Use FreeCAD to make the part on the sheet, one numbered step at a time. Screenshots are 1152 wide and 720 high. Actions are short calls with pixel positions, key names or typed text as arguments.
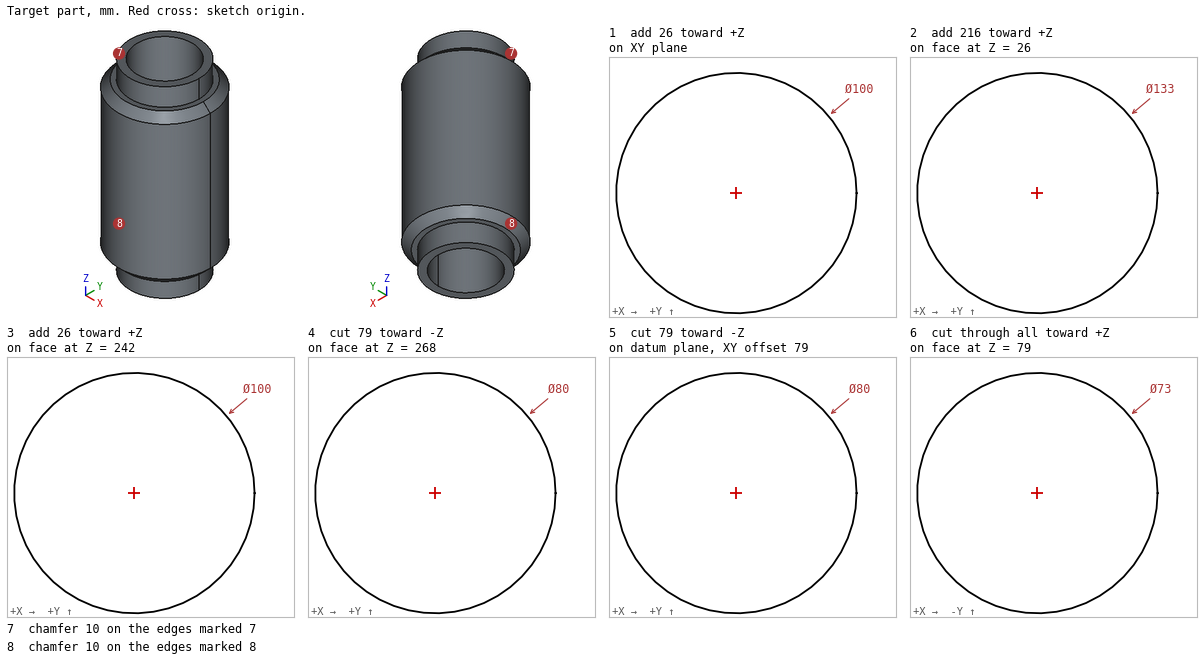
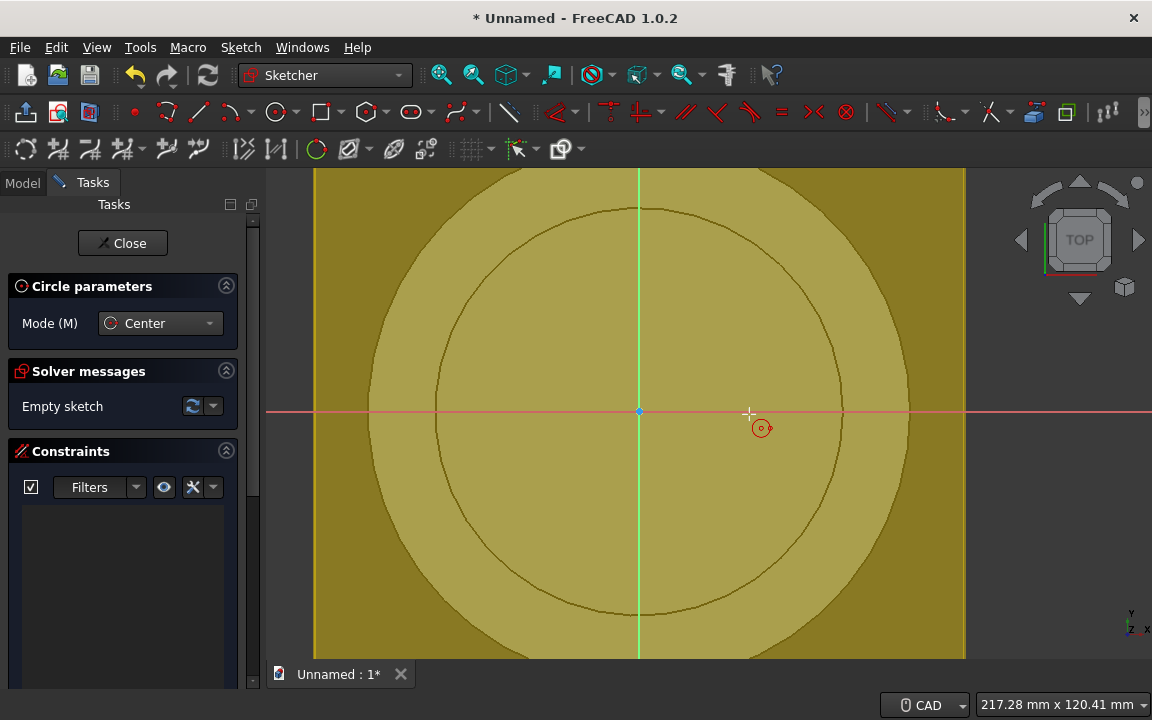
click(639, 412)
move(754, 296)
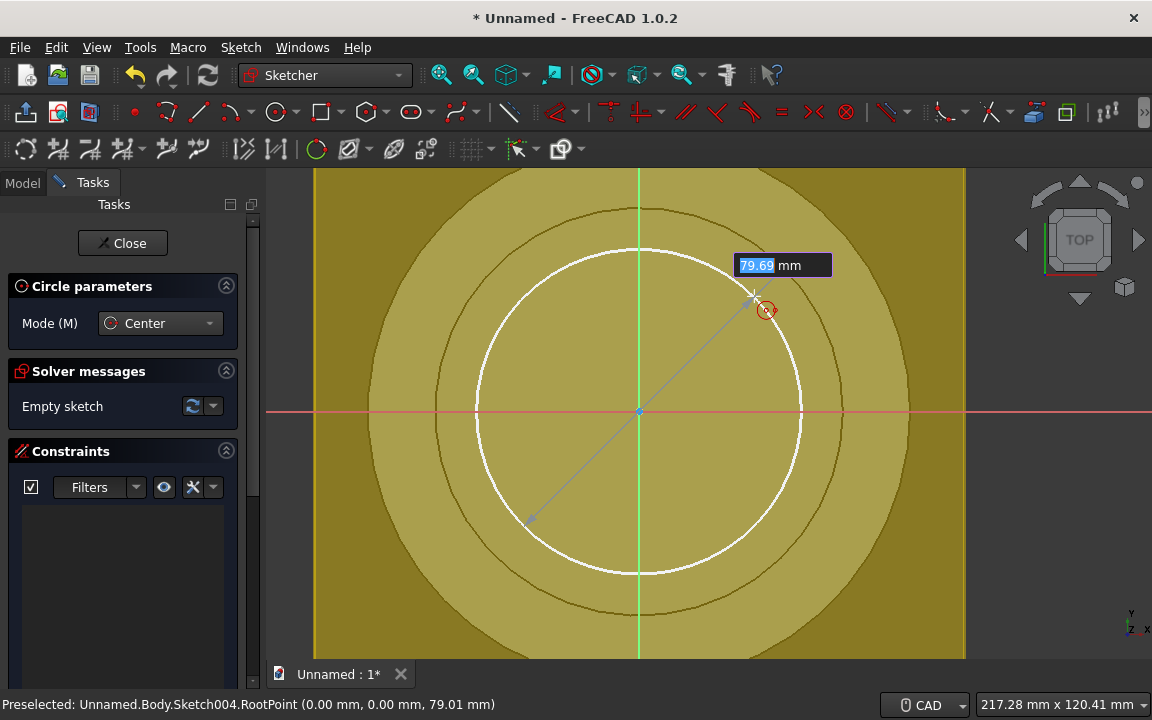
text(80)
key(Return)
key(Escape)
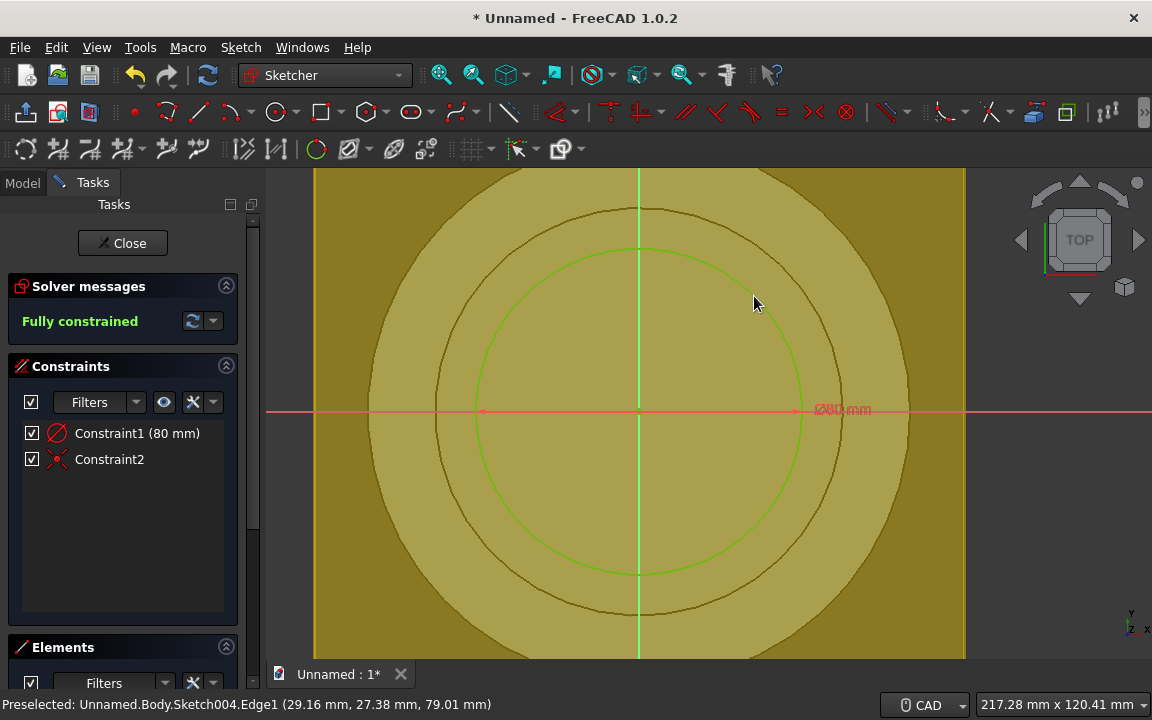
click(123, 243)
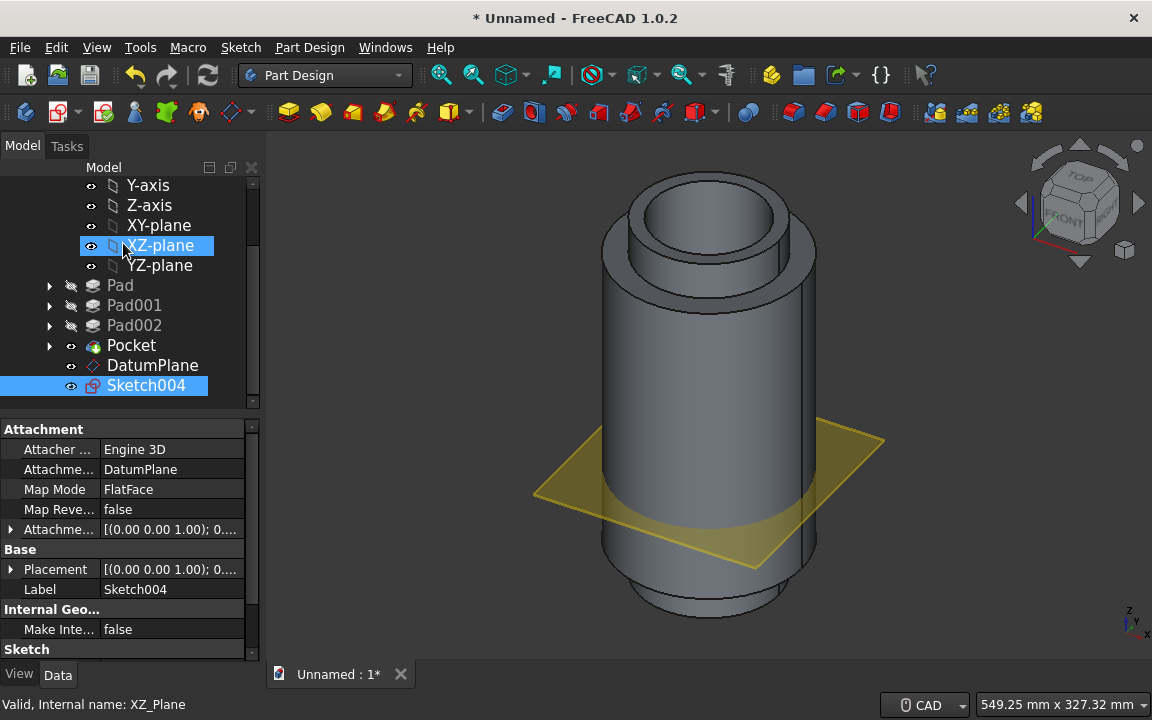
click(504, 112)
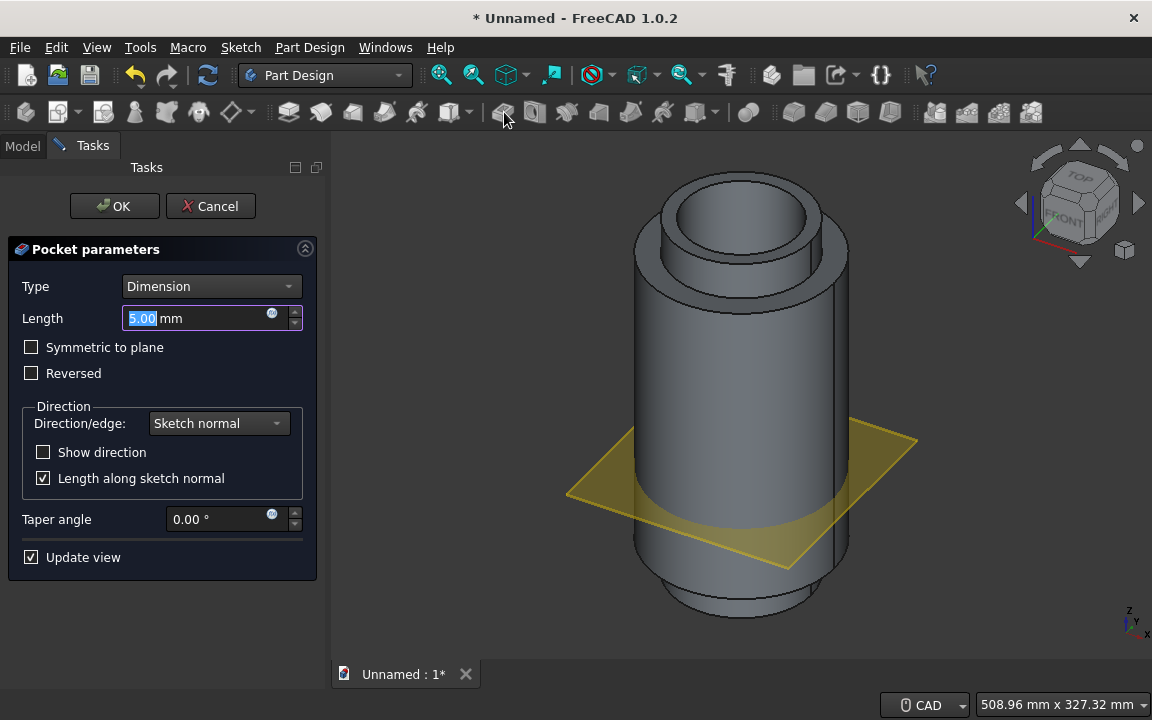
text(79)
key(Tab)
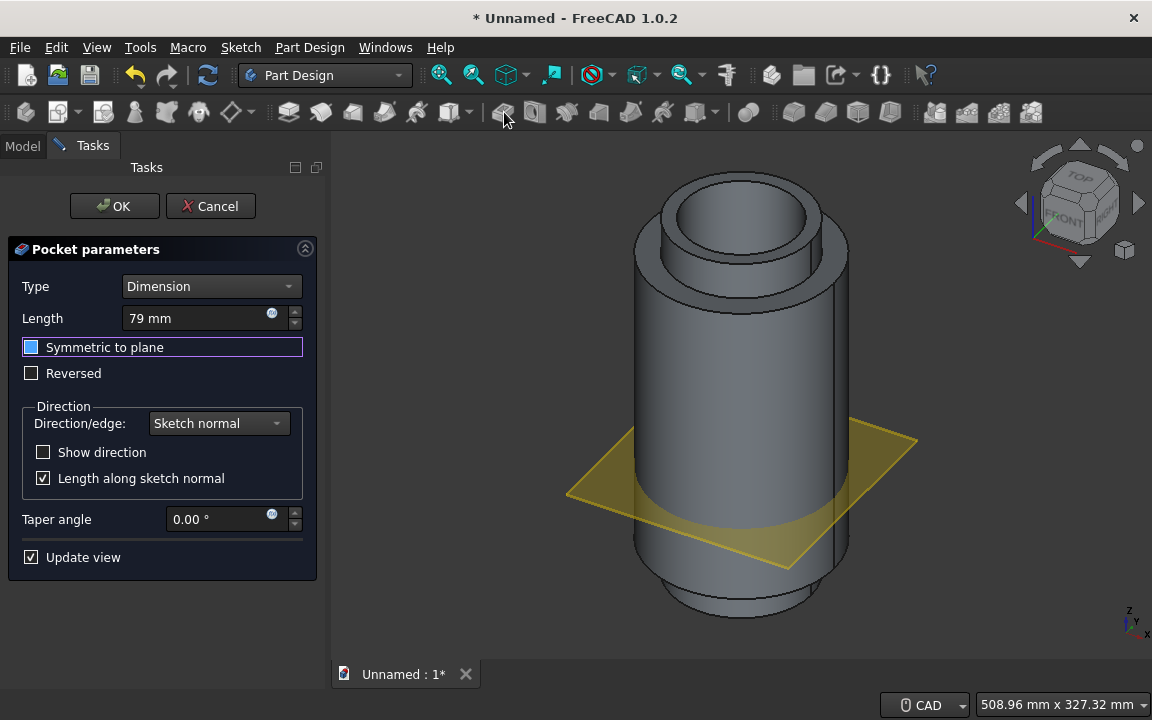
click(115, 206)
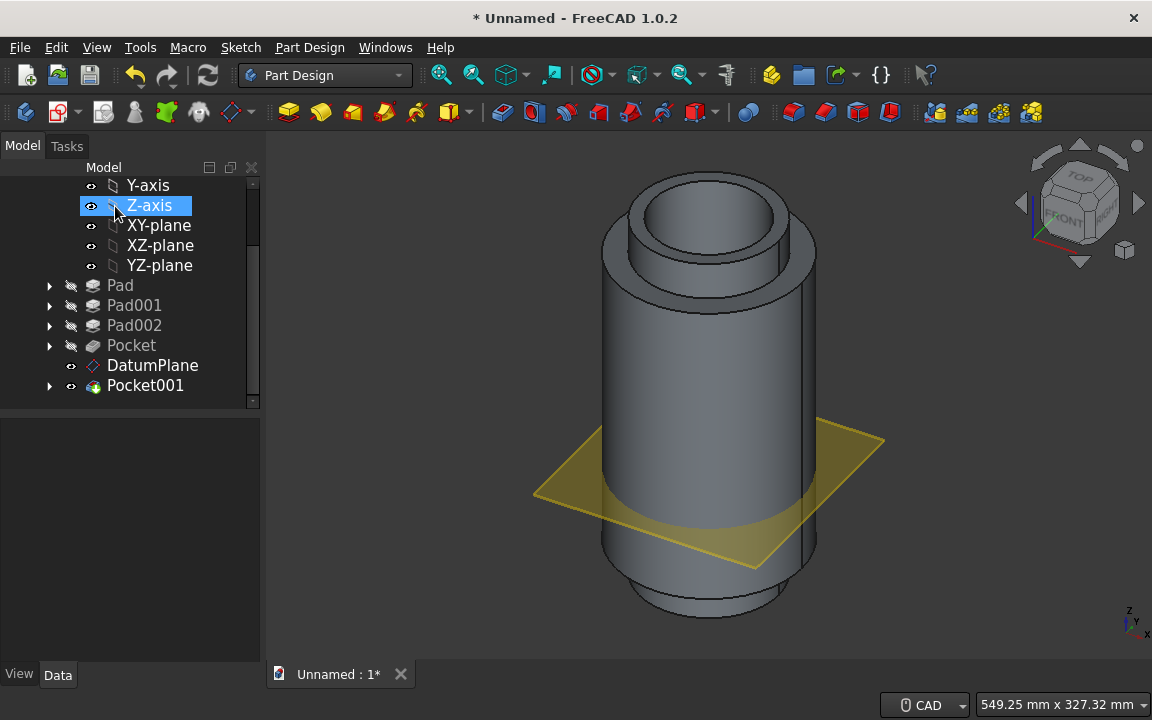
click(116, 366)
key(space)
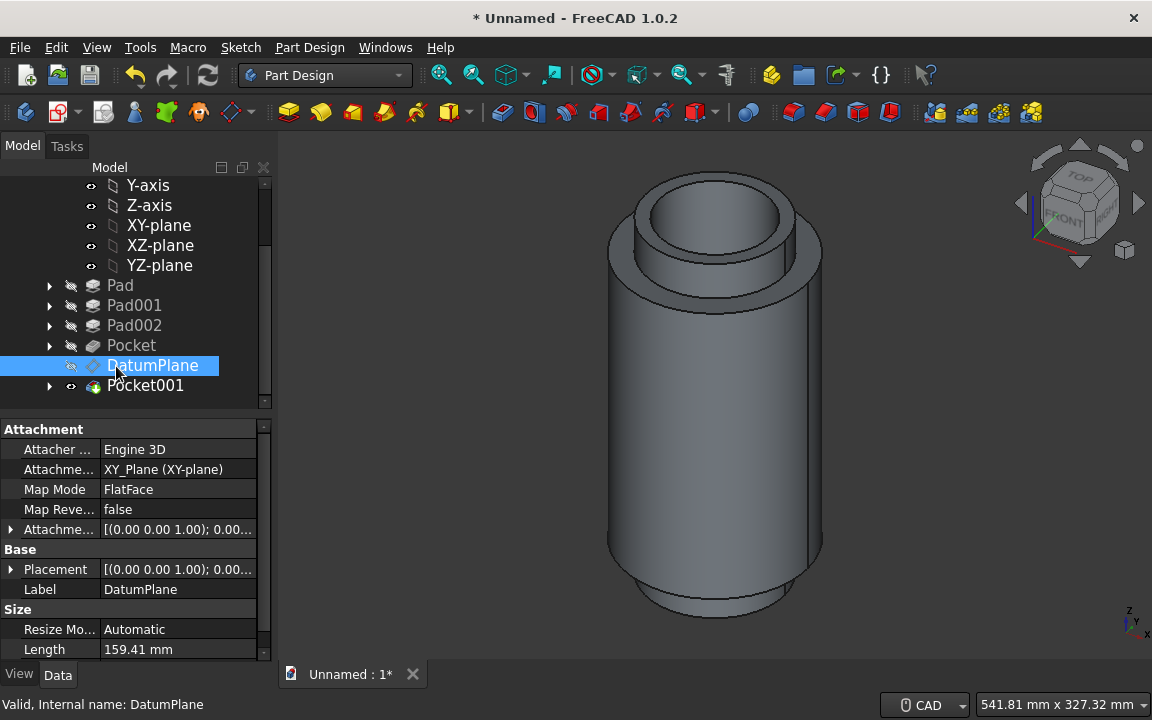
key(5)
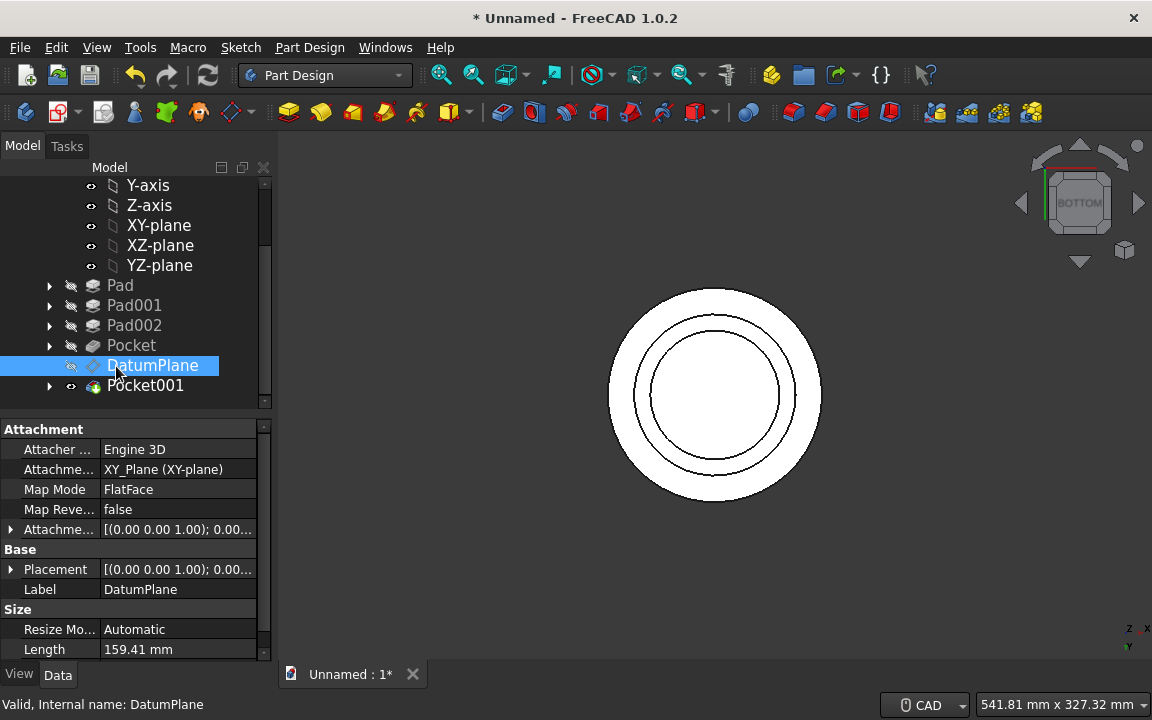
click(442, 76)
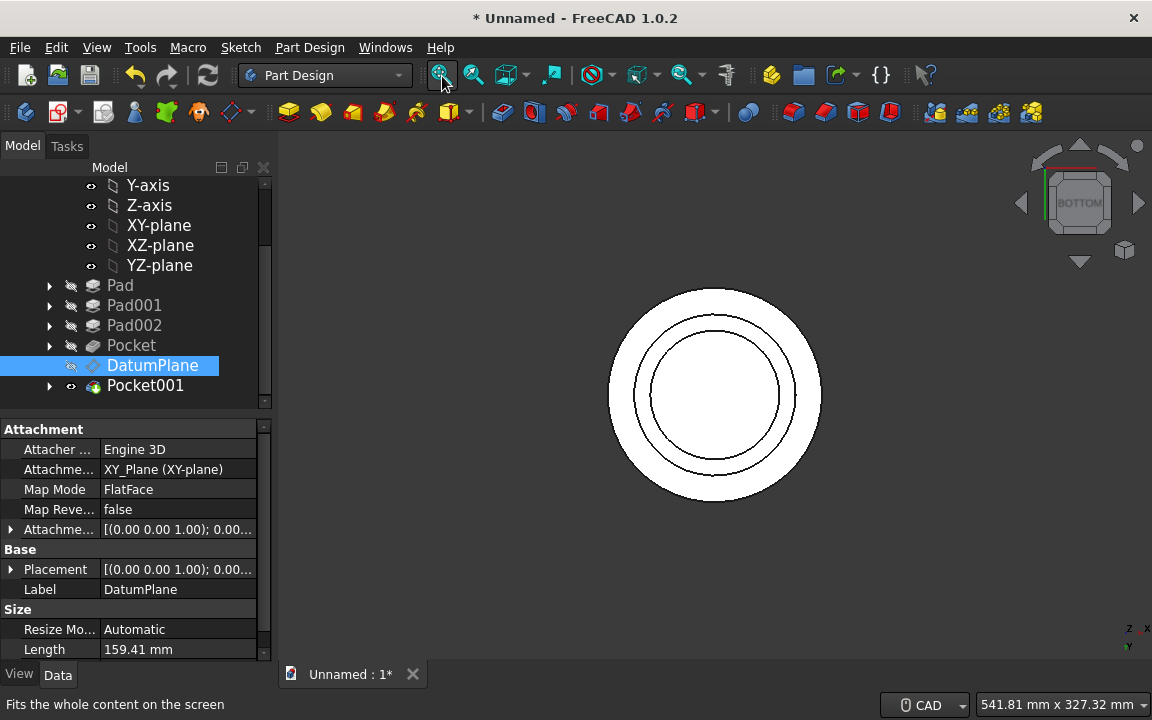
click(715, 394)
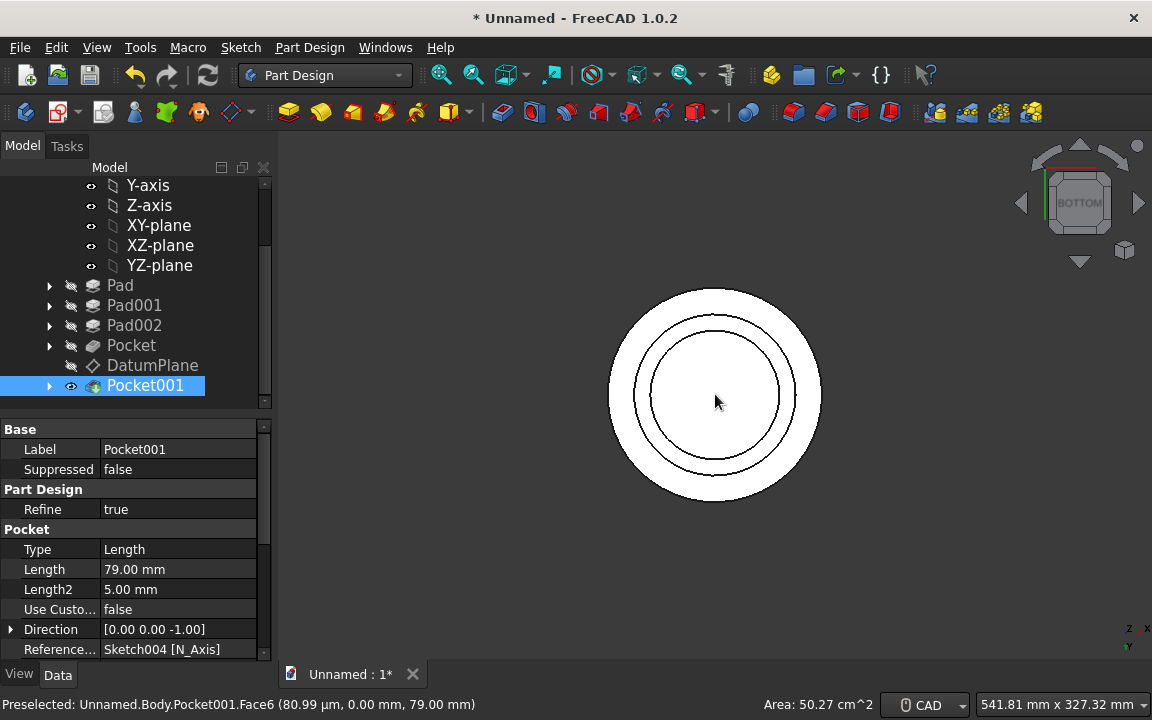
click(58, 112)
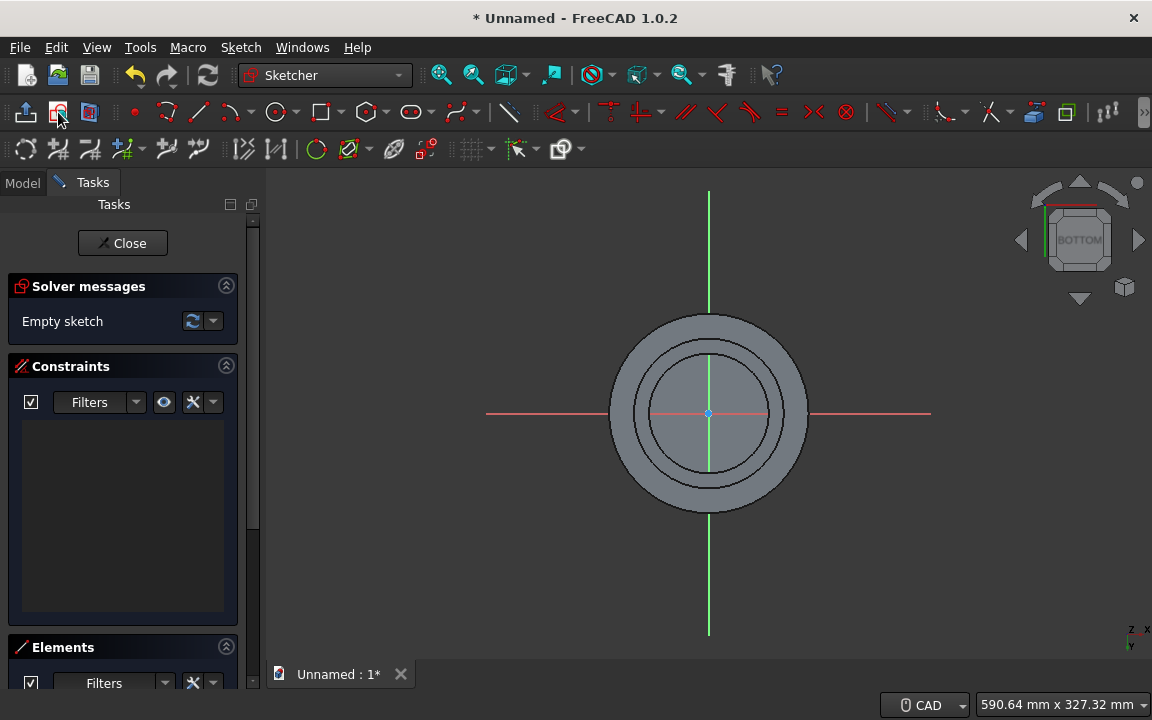
key(q)
key(s)